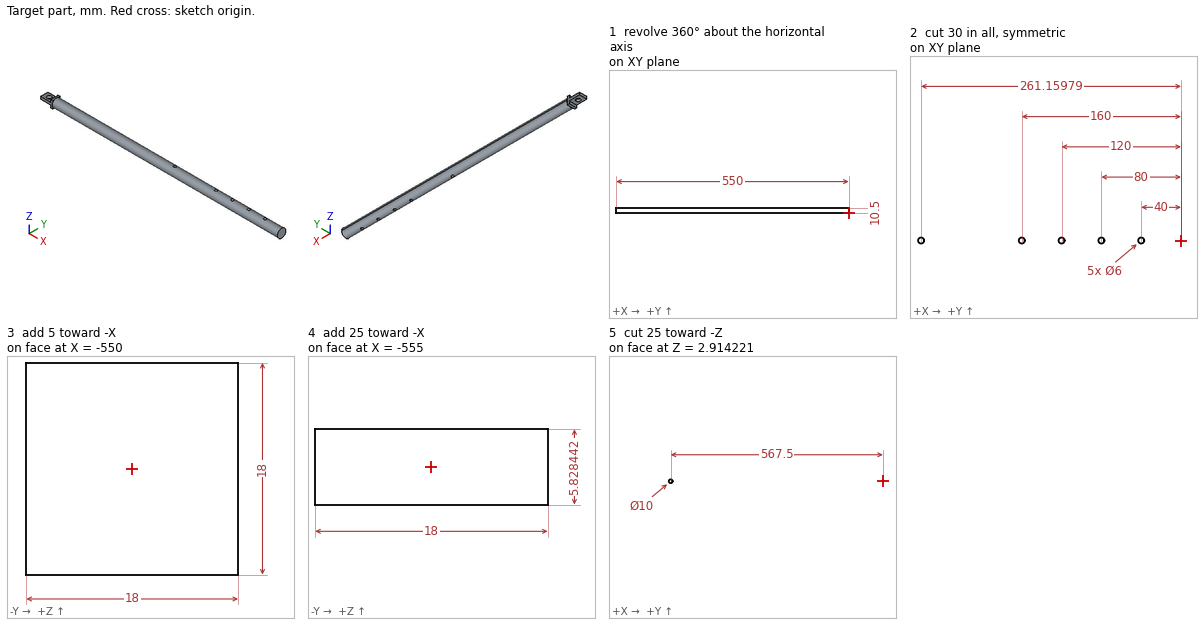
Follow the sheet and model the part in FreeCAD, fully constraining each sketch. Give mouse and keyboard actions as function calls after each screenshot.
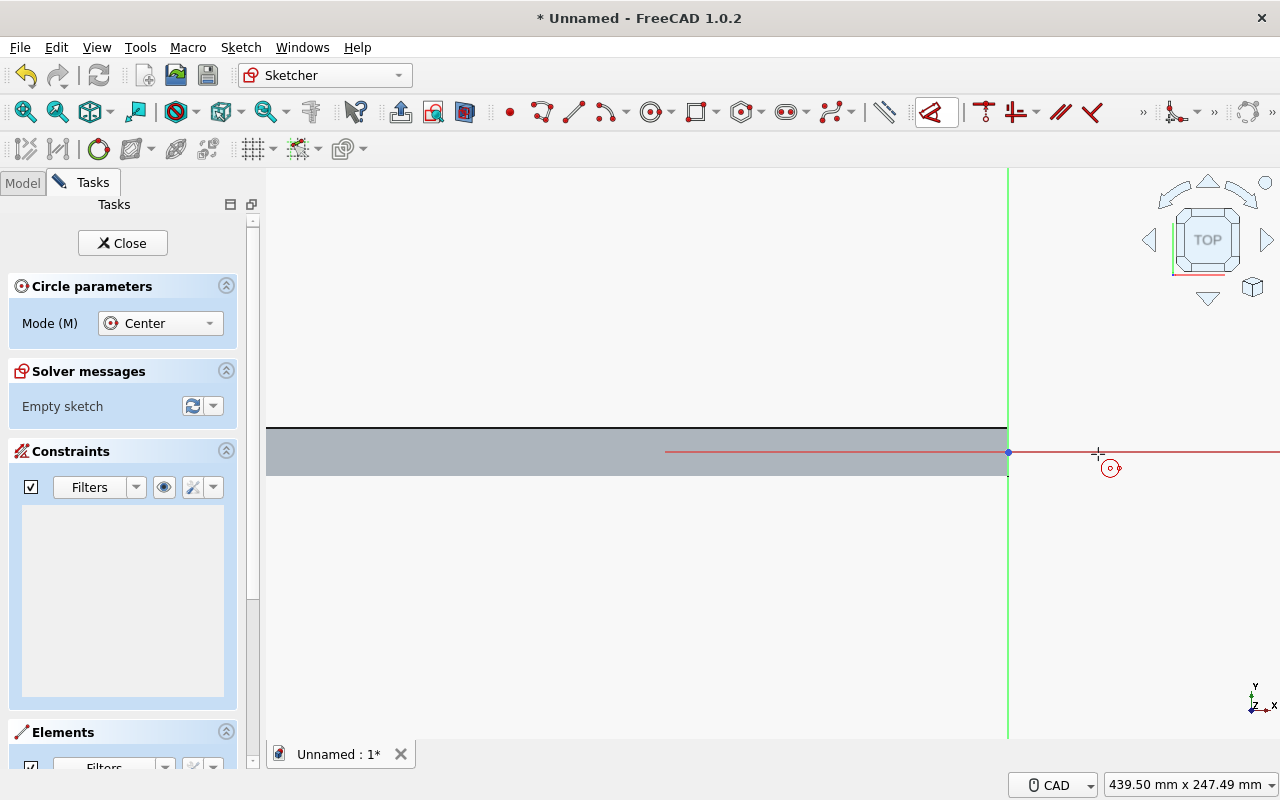
scroll(916, 452, up, 6)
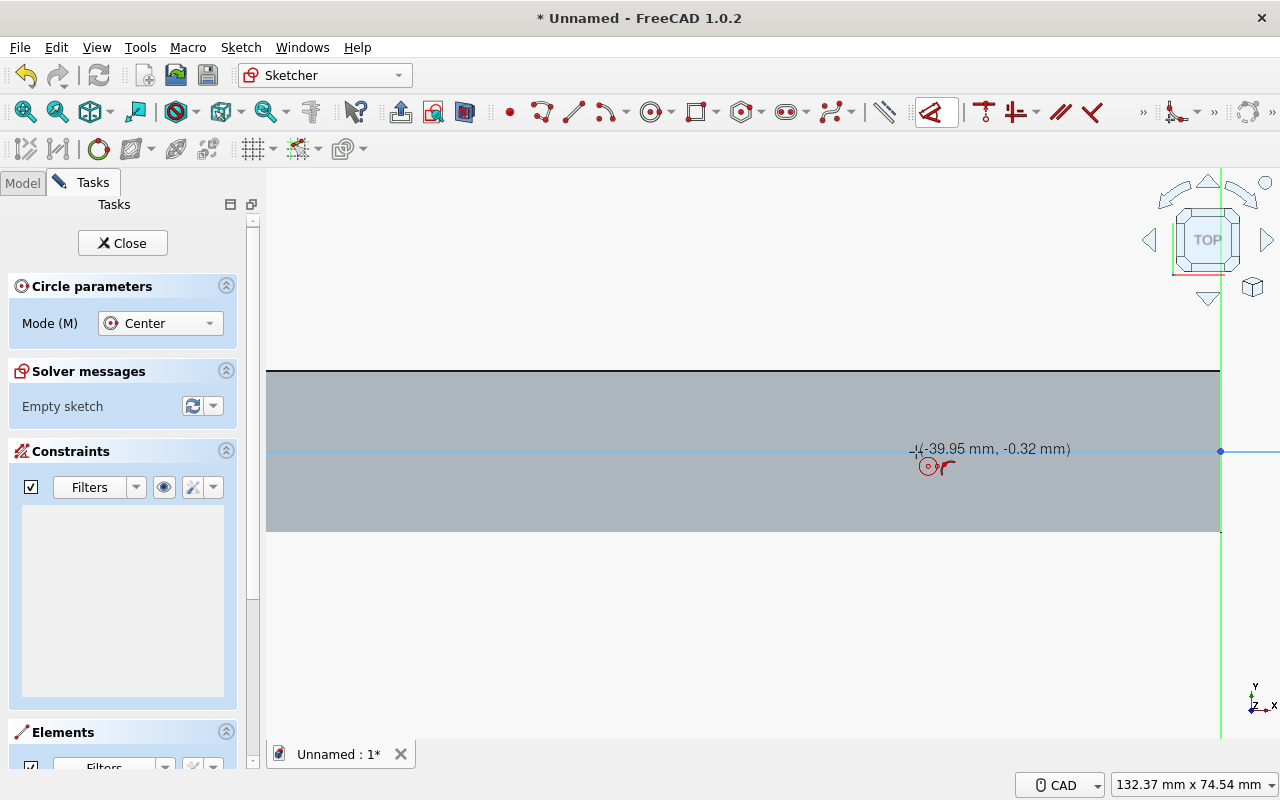
click(914, 452)
click(930, 435)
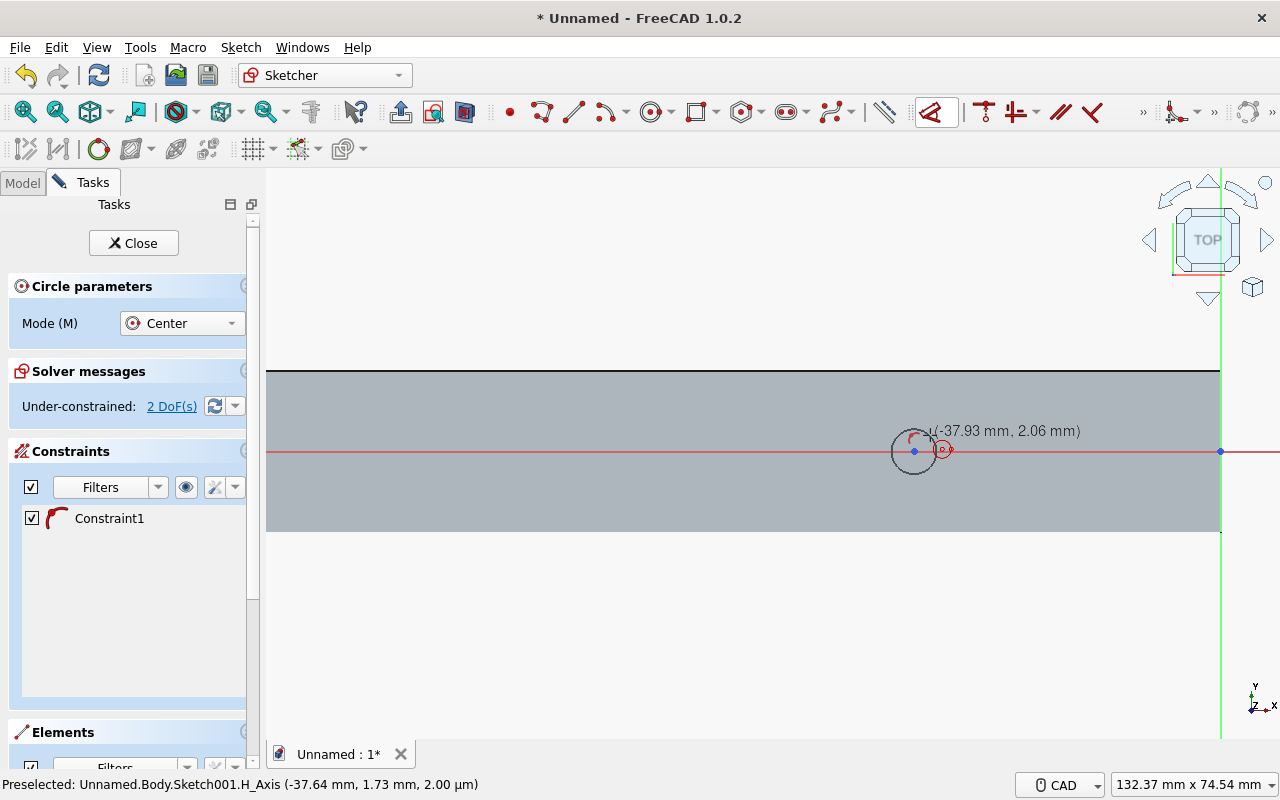
click(608, 452)
click(624, 435)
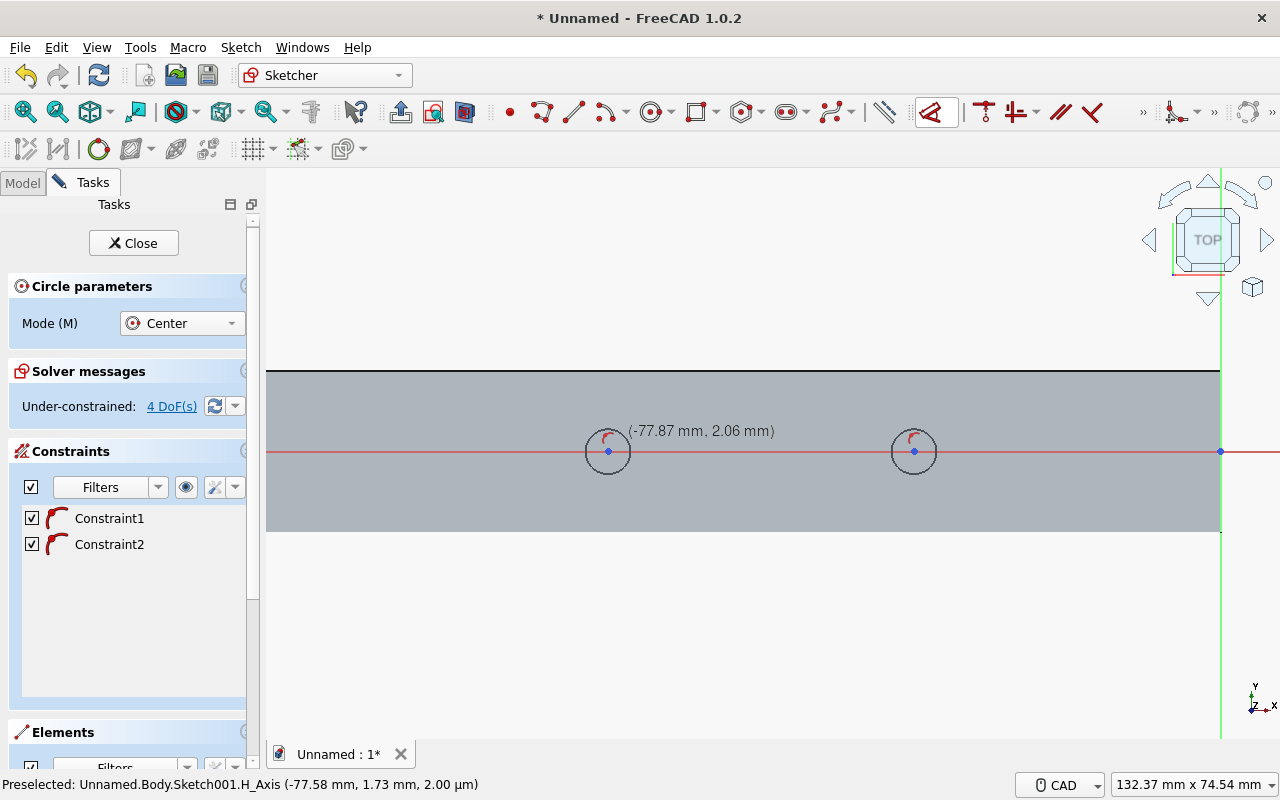
click(301, 452)
click(318, 435)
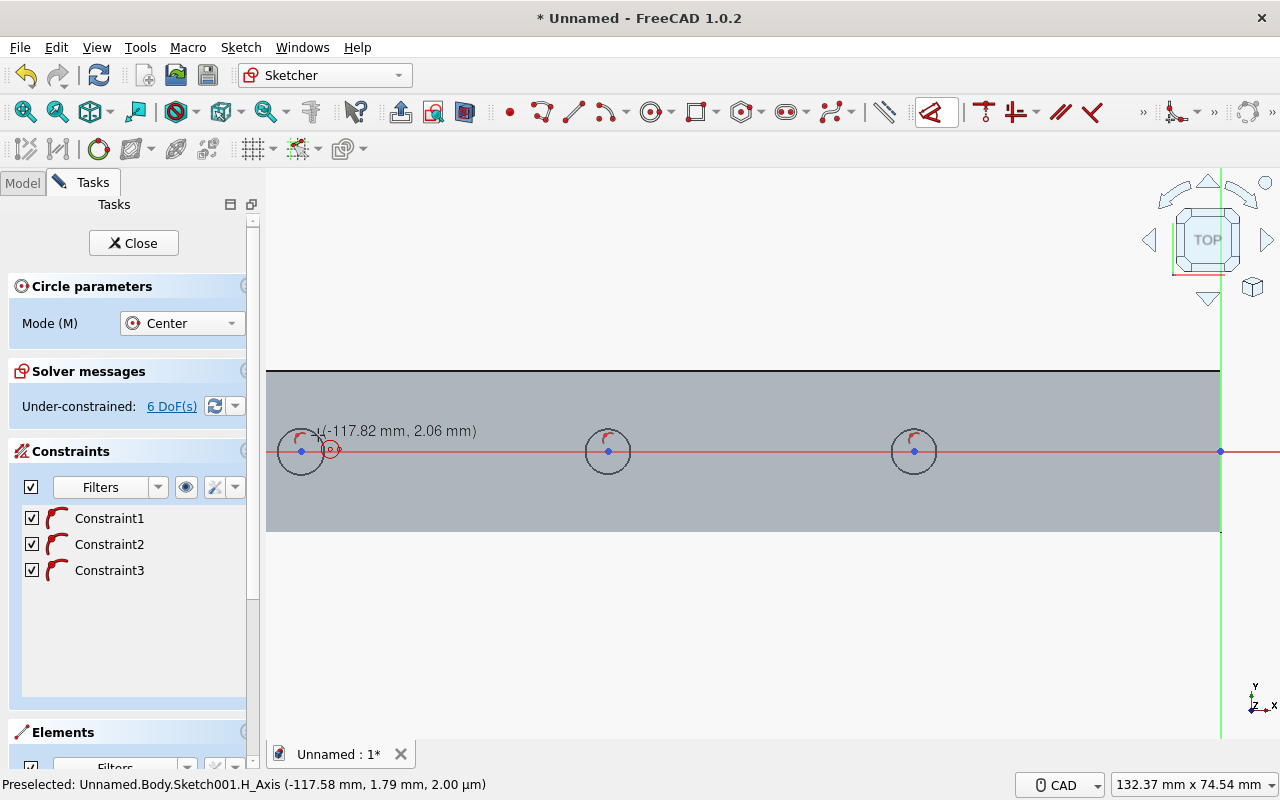
scroll(918, 454, down, 6)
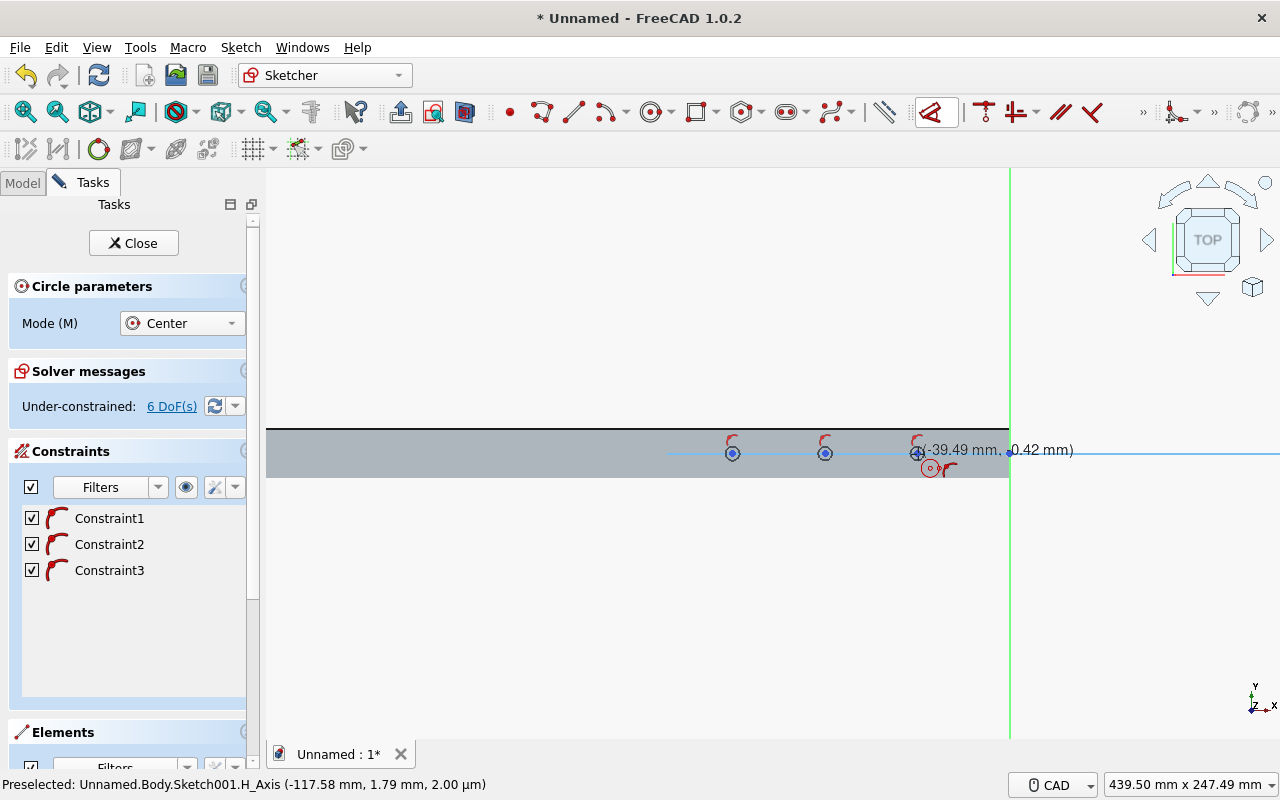
scroll(640, 454, up, 6)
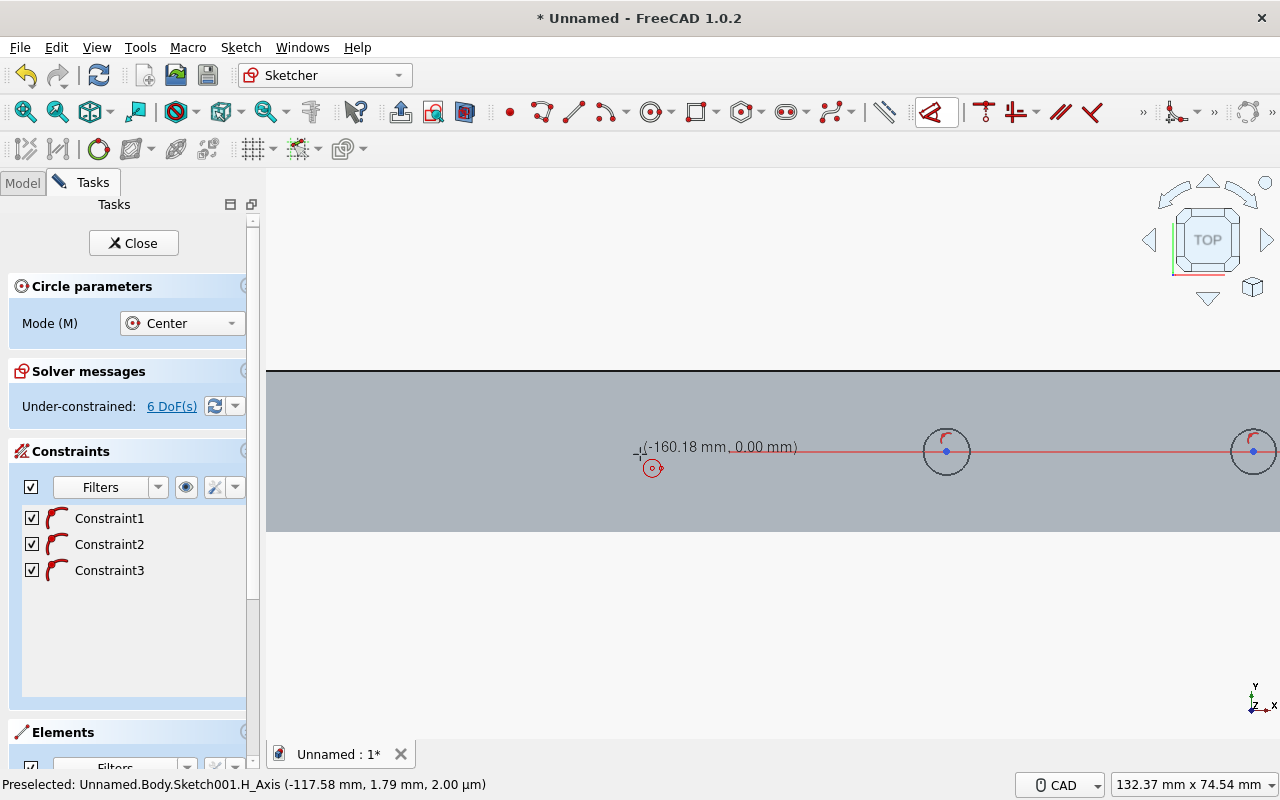
click(641, 452)
click(657, 435)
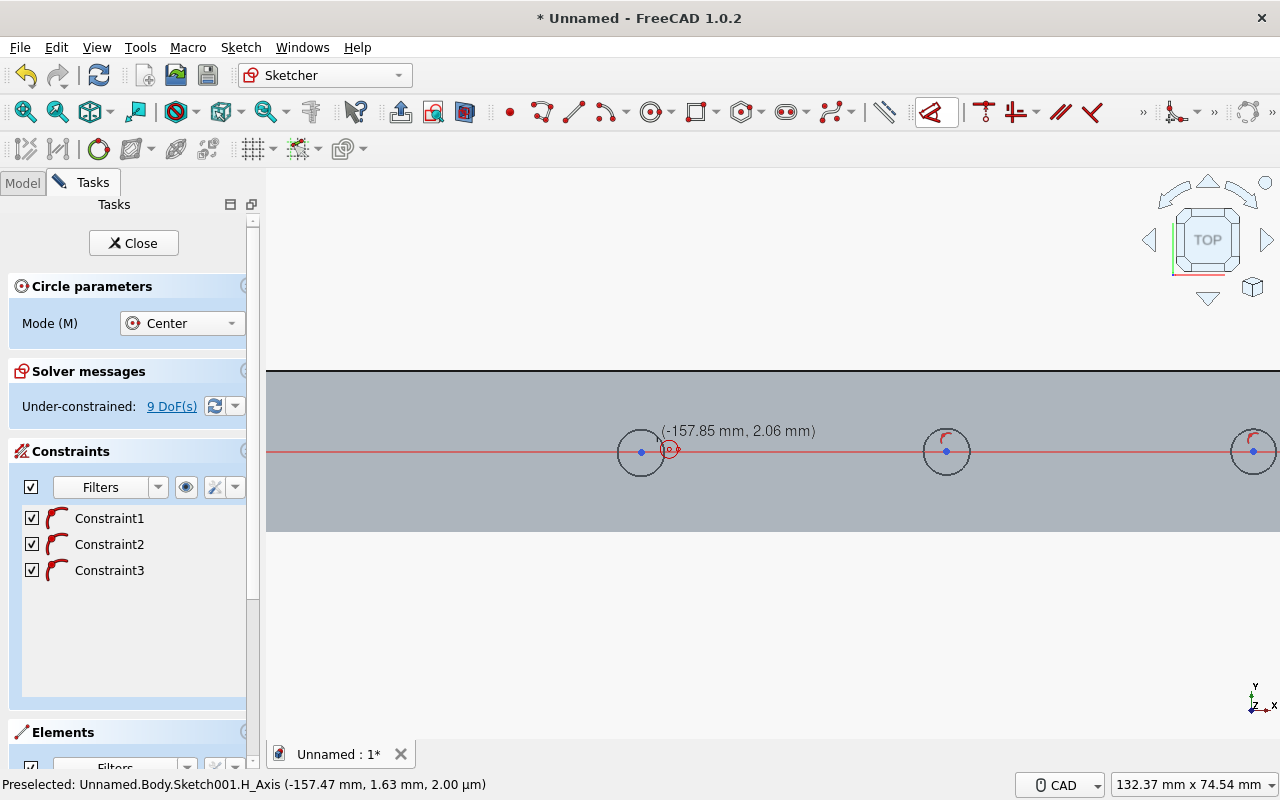
scroll(640, 454, down, 6)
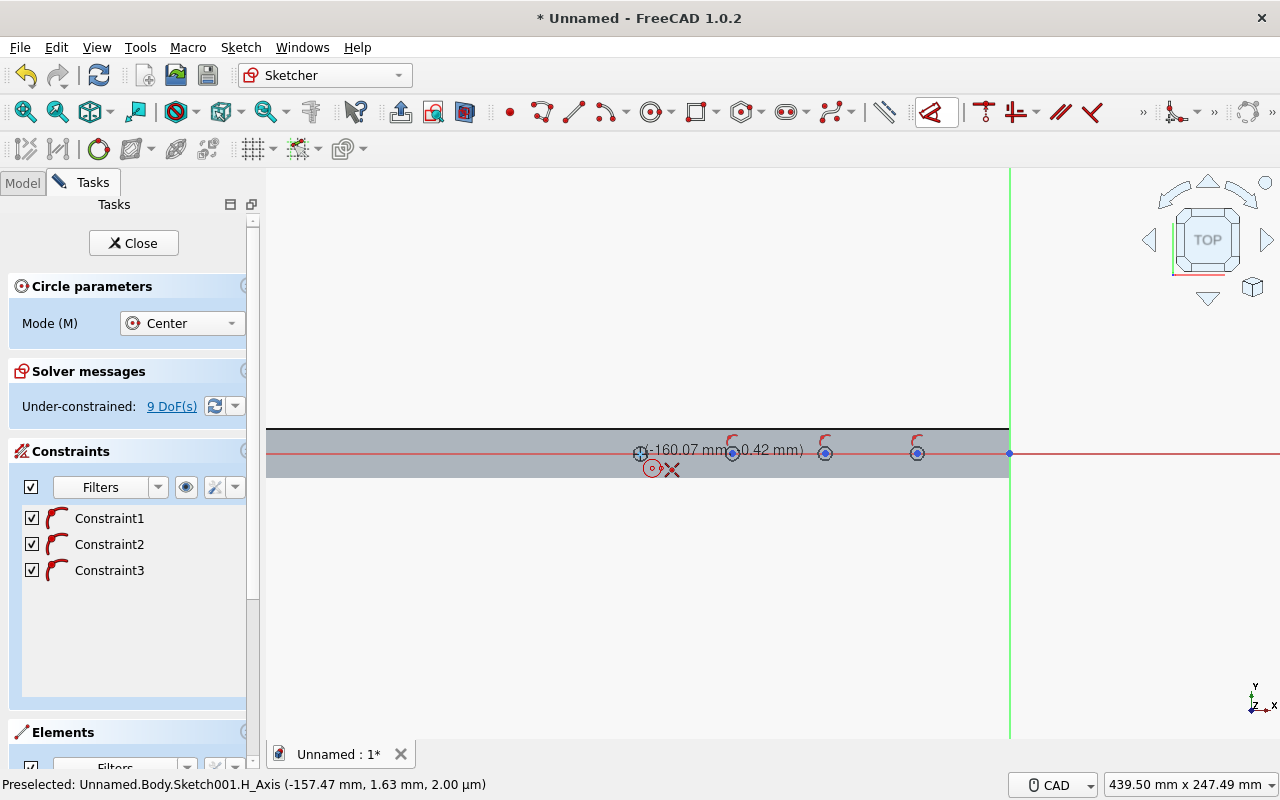
scroll(407, 454, up, 6)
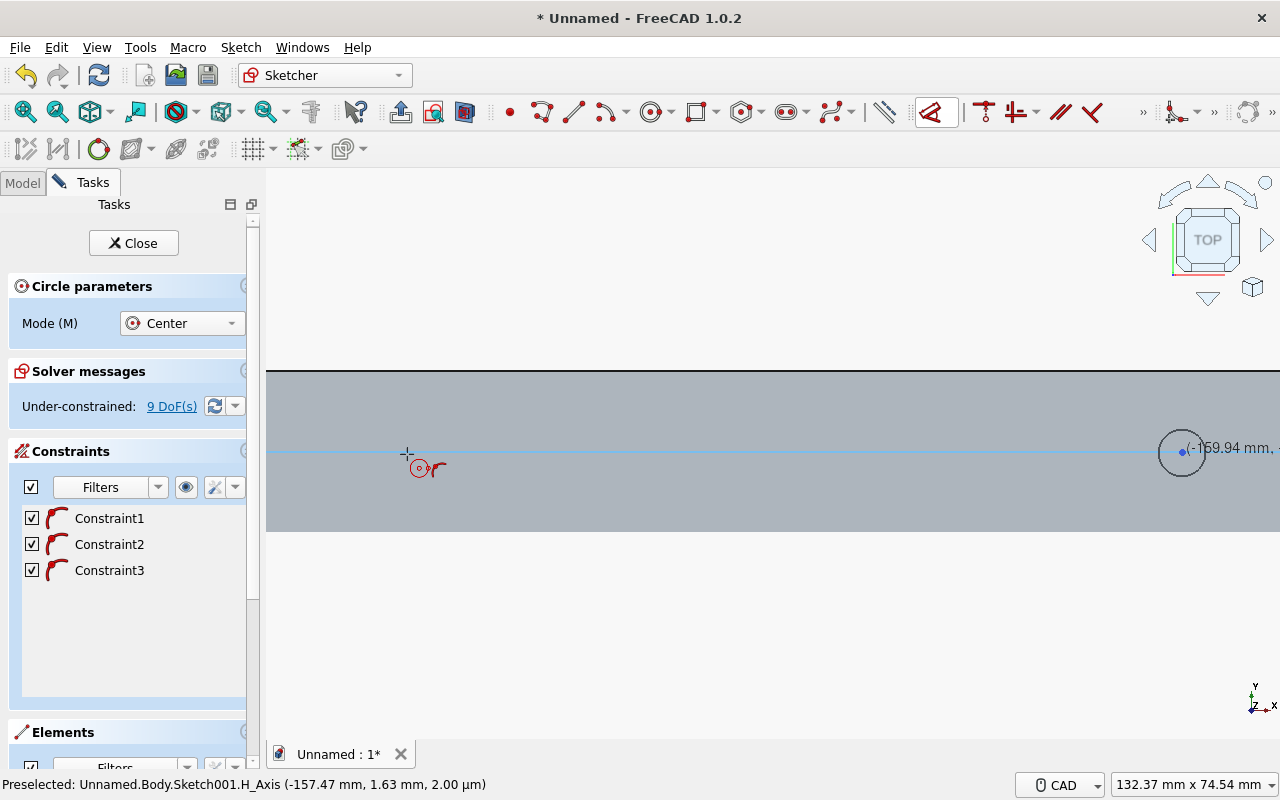
click(407, 452)
click(423, 435)
key(Escape)